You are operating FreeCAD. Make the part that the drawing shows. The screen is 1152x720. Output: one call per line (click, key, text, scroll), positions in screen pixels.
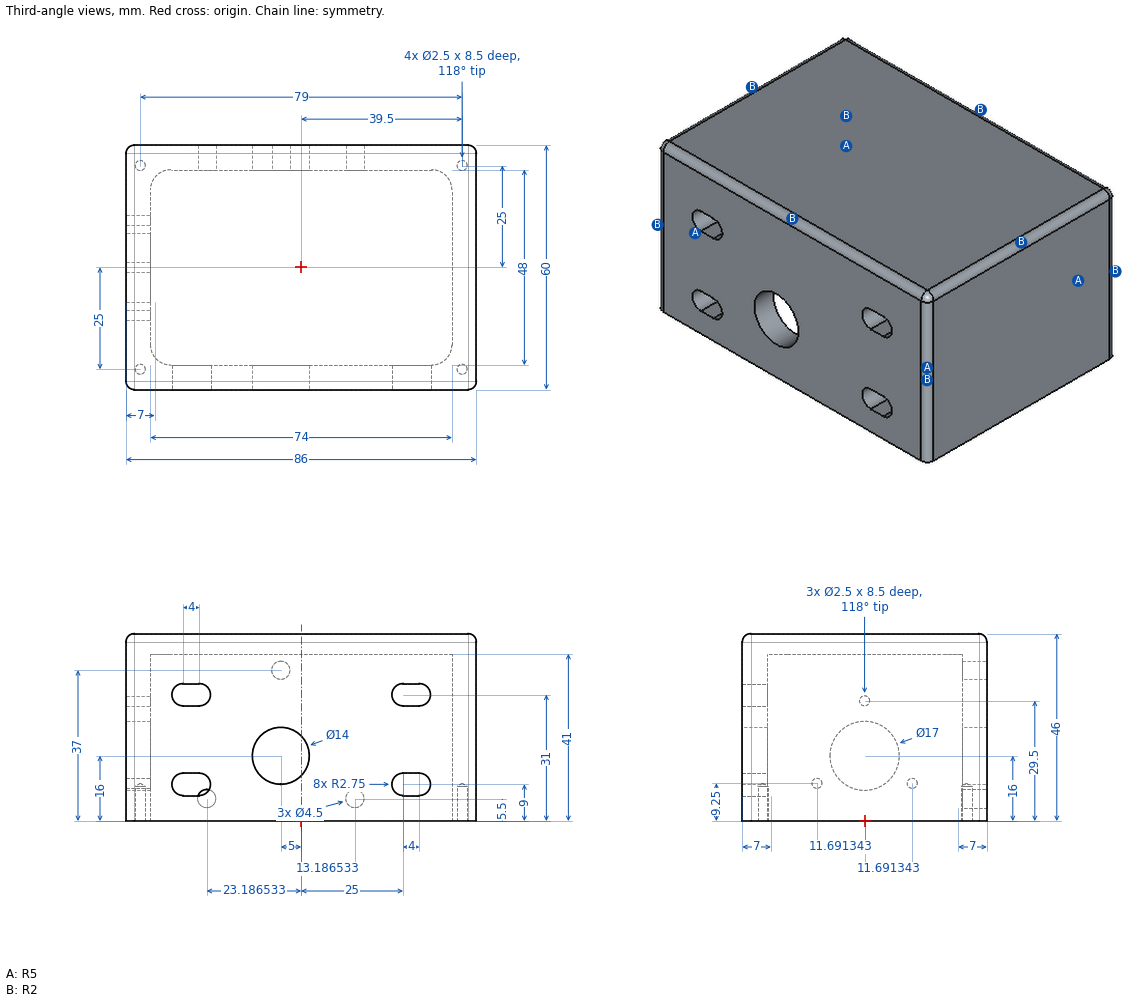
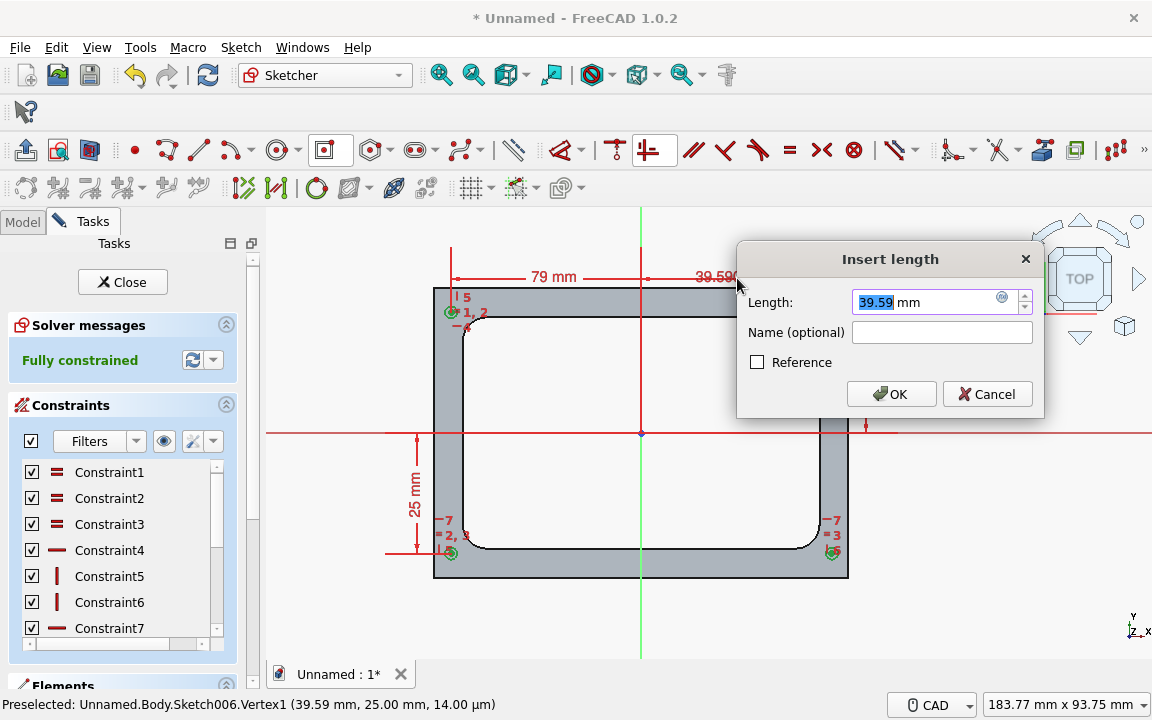
text(39.5)
key(Return)
key(Escape)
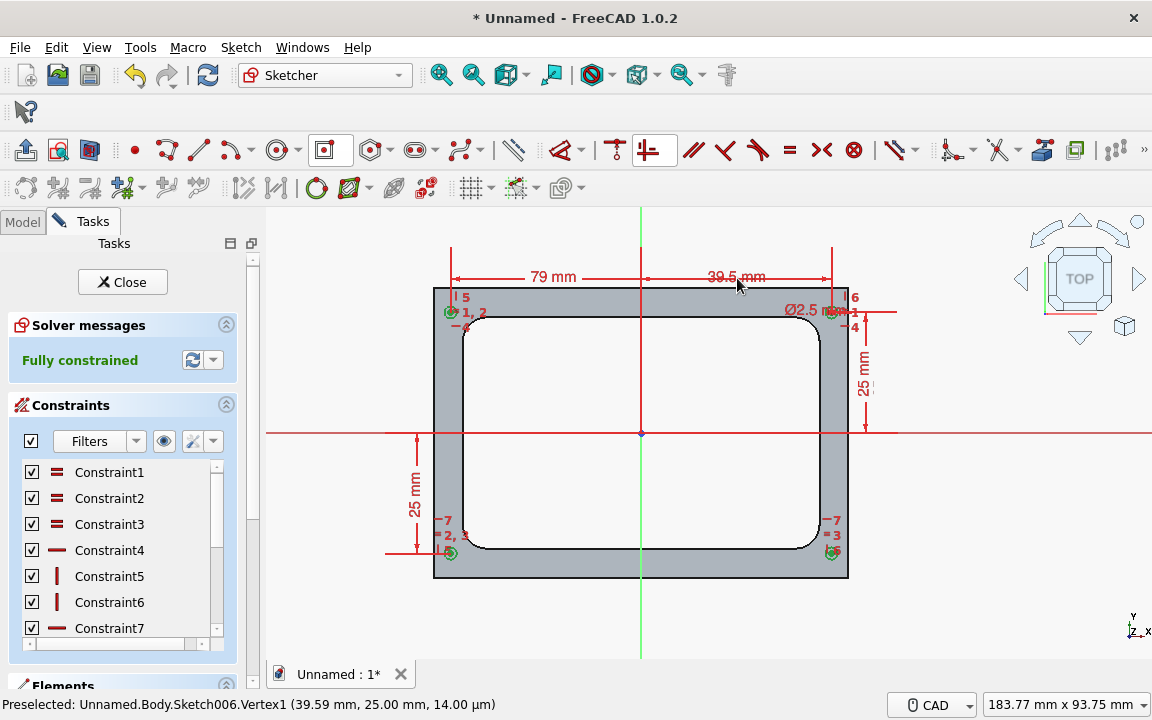
click(123, 282)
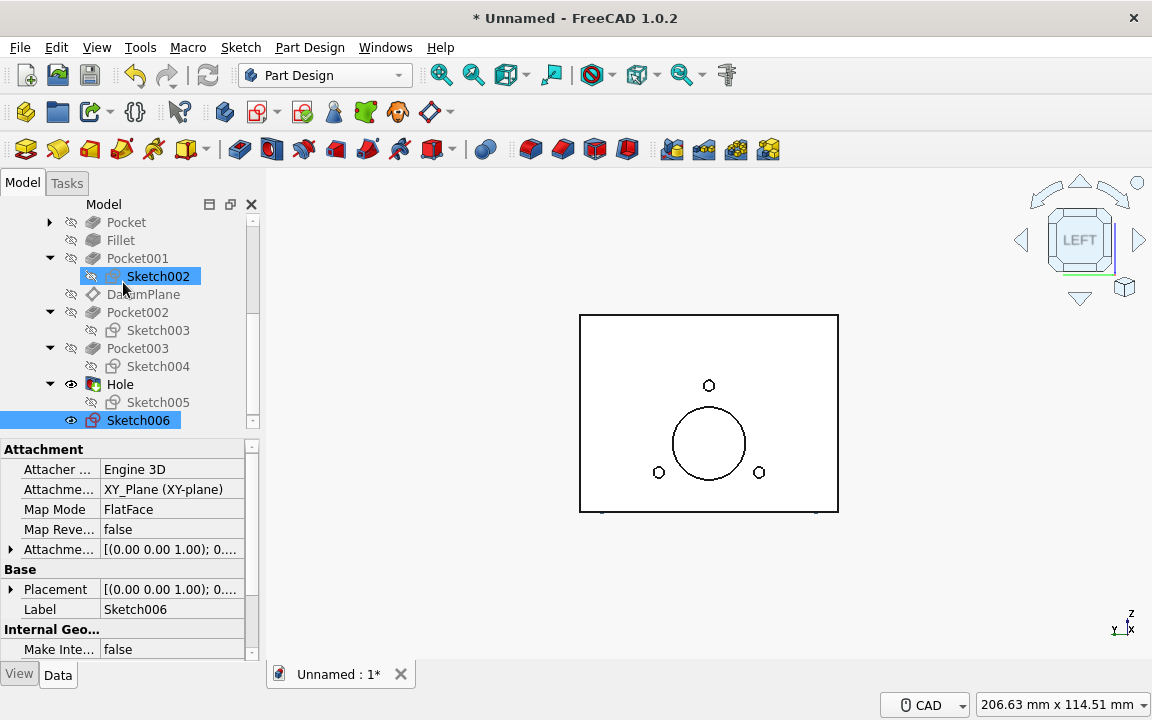
click(272, 150)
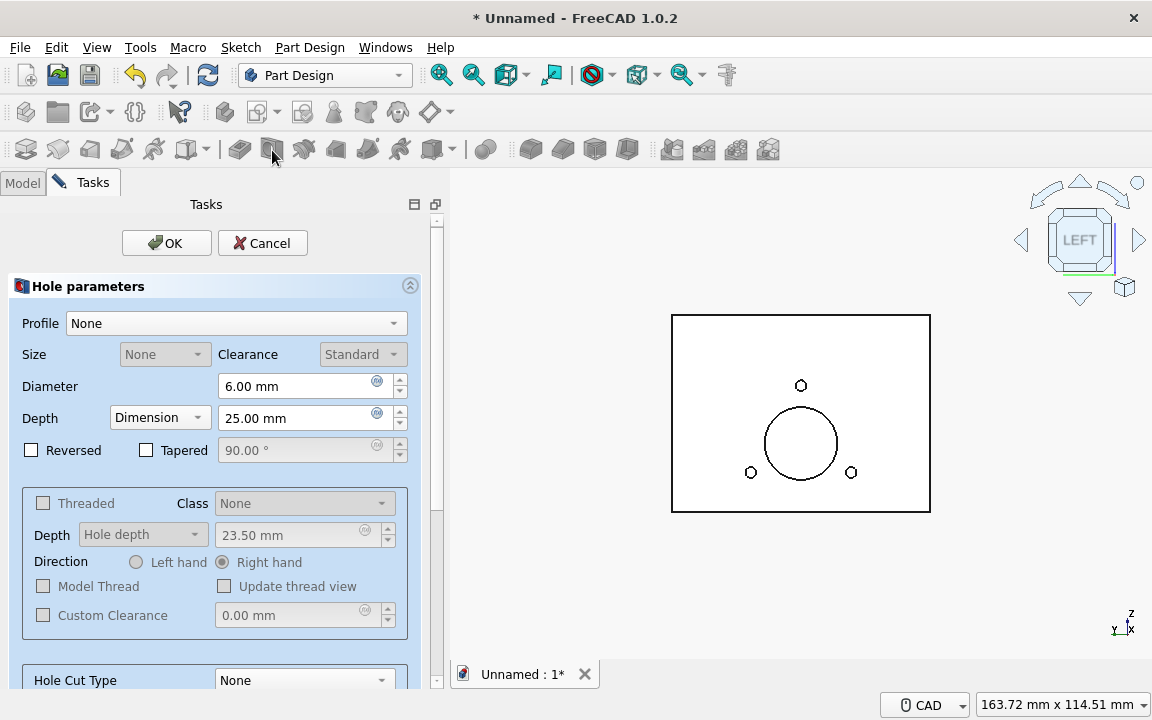
triple_click(305, 386)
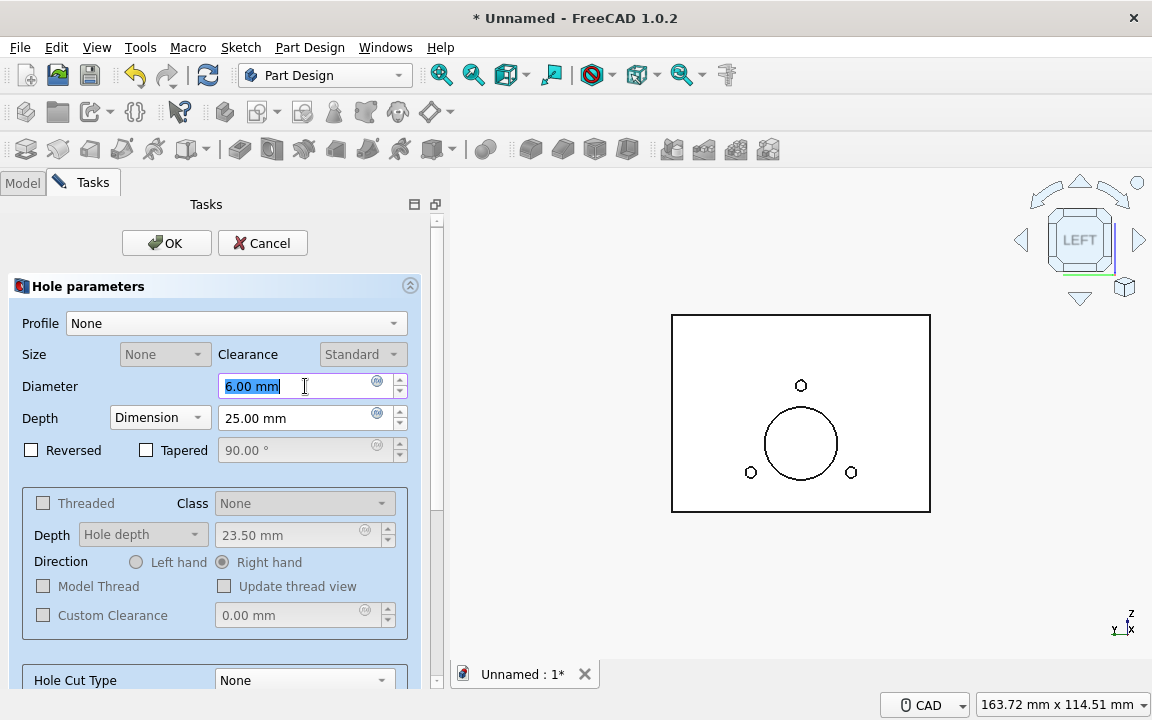
text(2.5)
key(Tab)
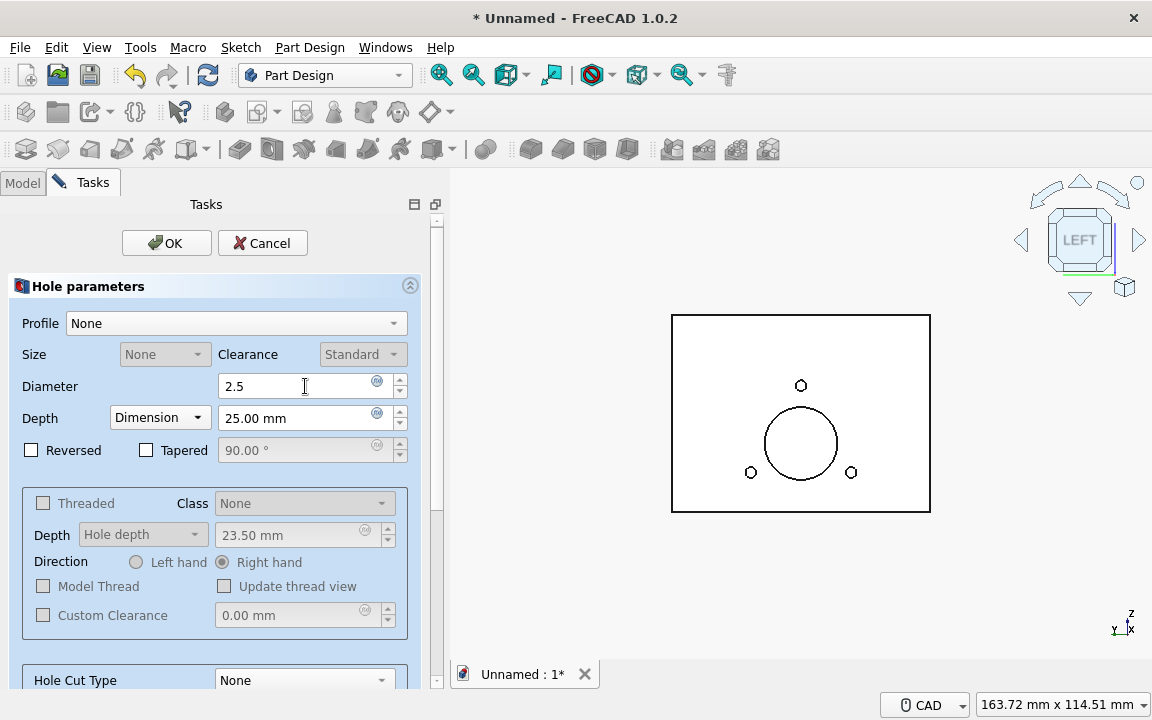
triple_click(305, 418)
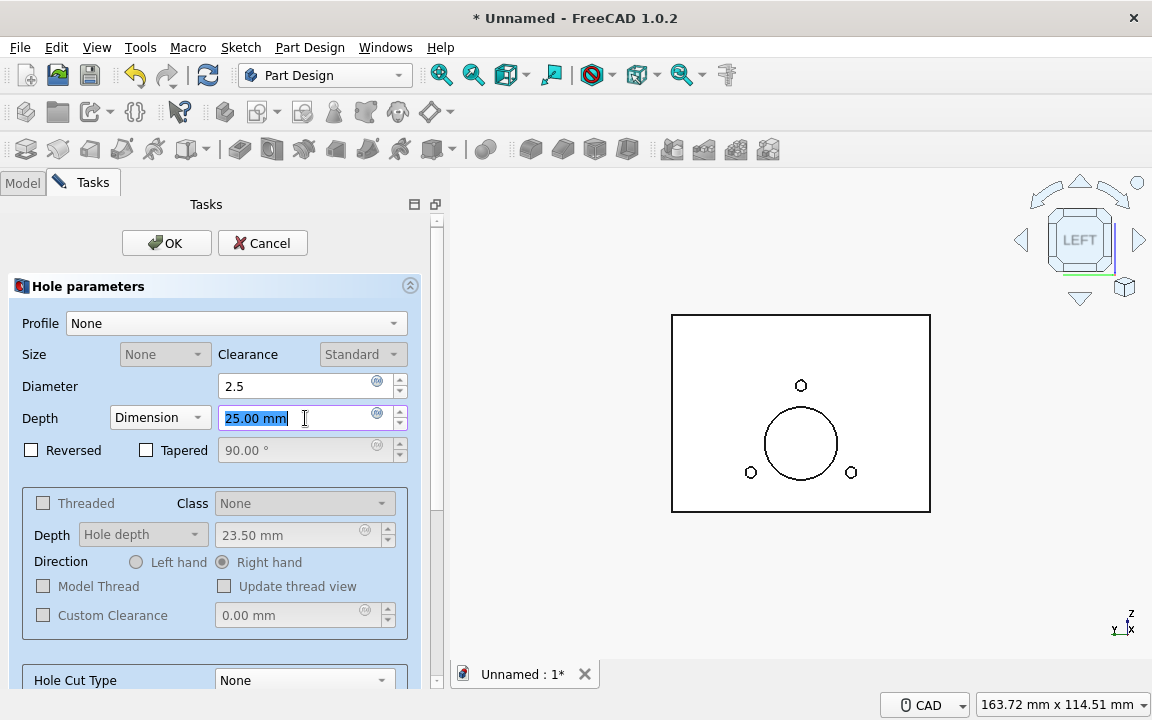
text(8.5)
key(Tab)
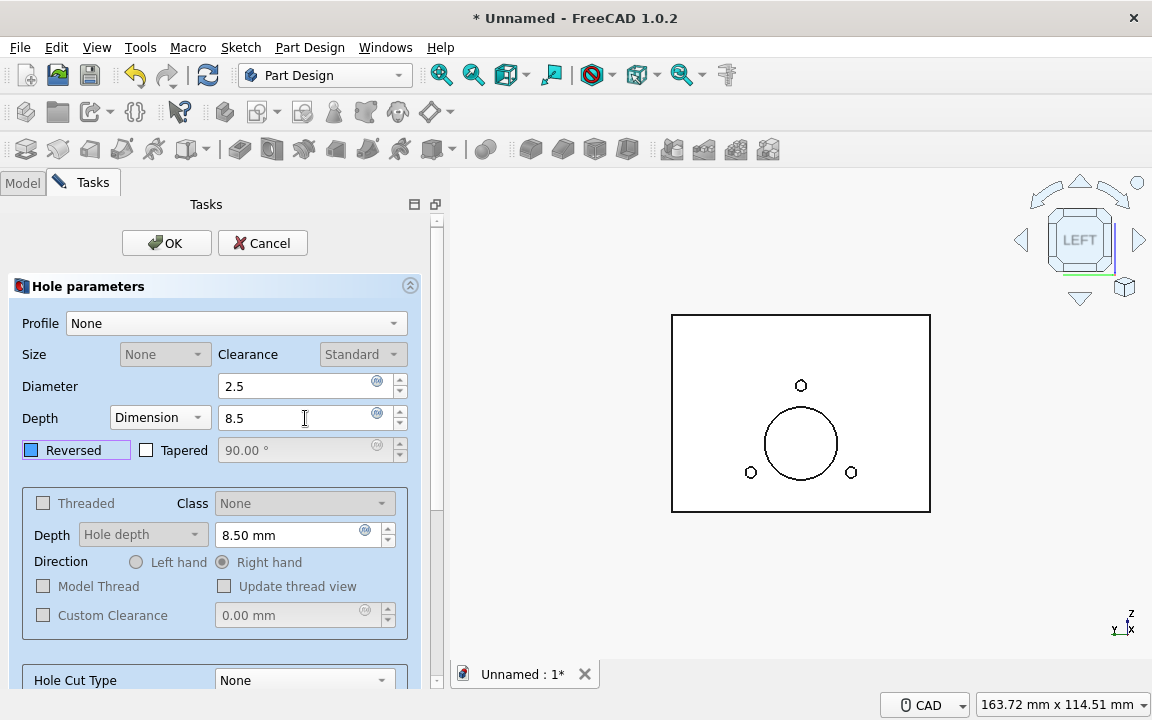
click(30, 450)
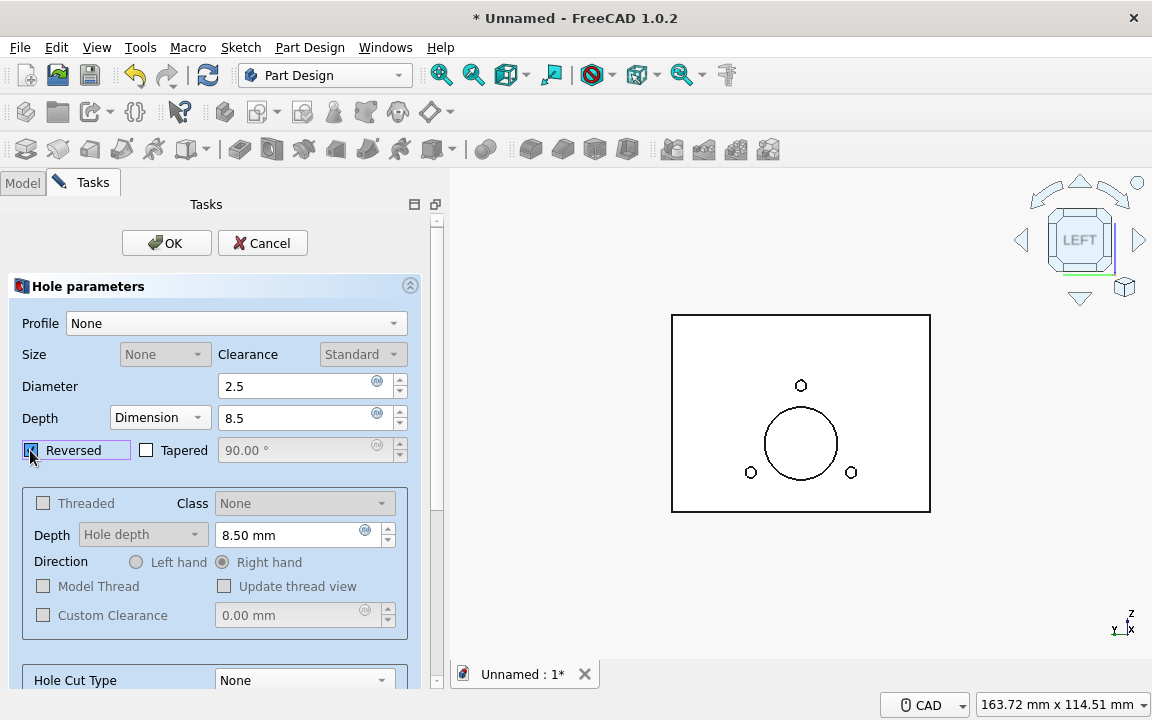
click(167, 243)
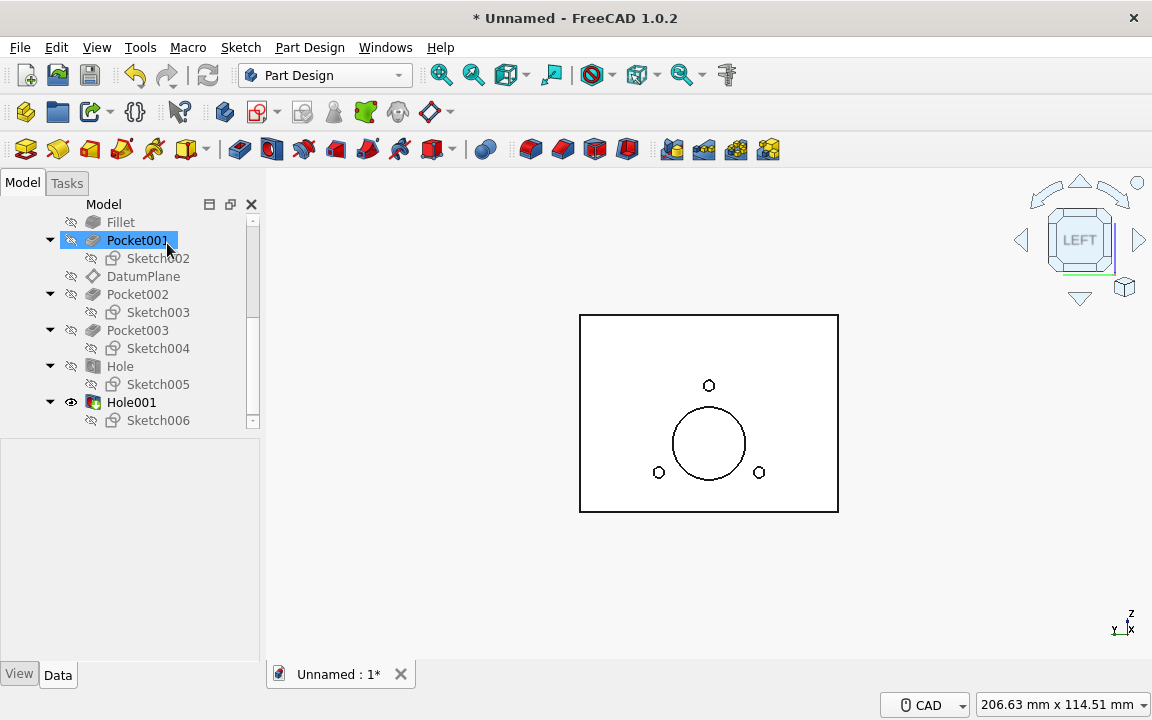
click(442, 76)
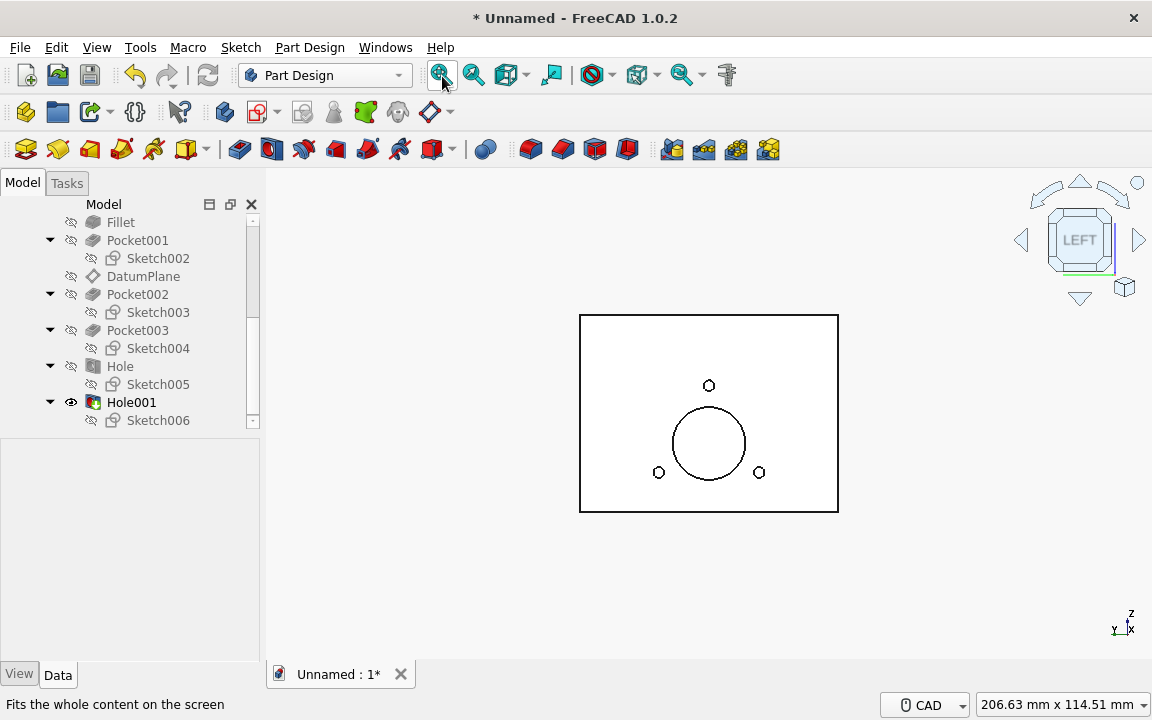
click(838, 412)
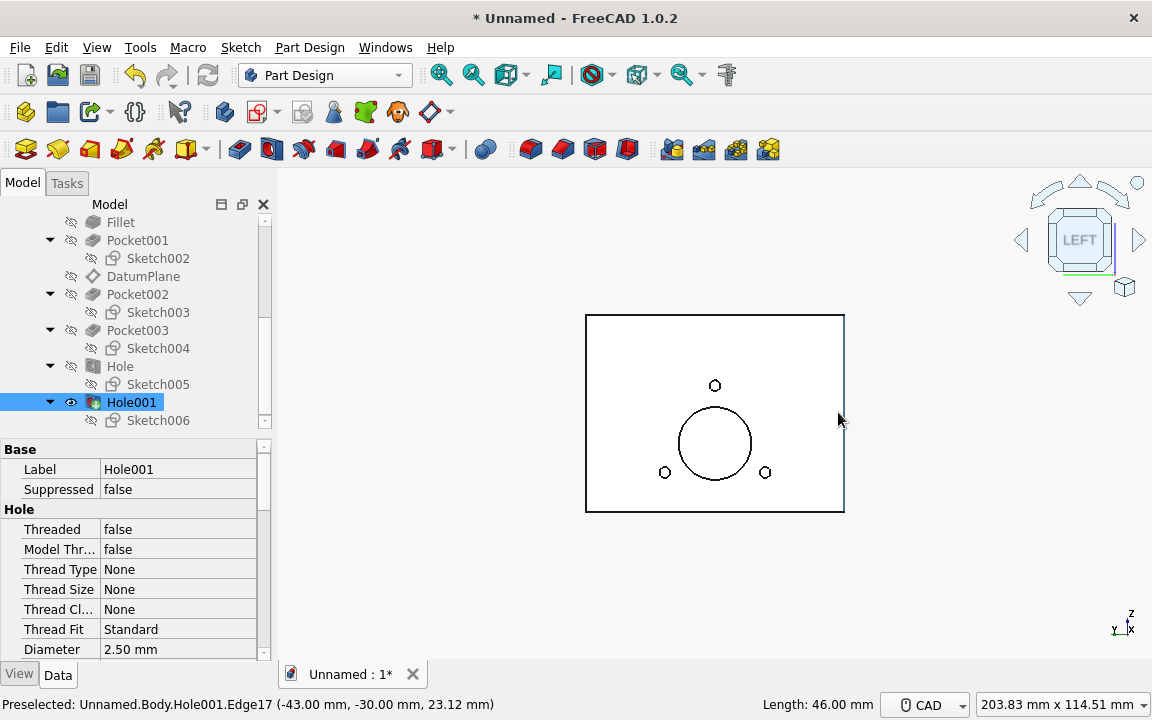
click(586, 412, ctrl)